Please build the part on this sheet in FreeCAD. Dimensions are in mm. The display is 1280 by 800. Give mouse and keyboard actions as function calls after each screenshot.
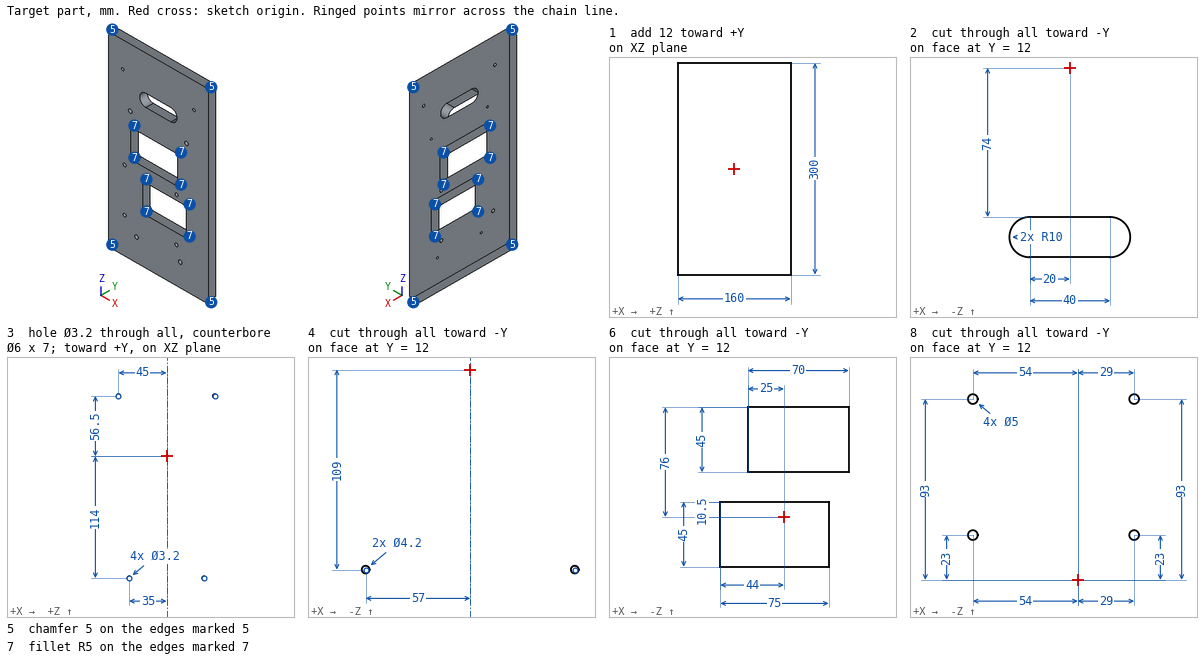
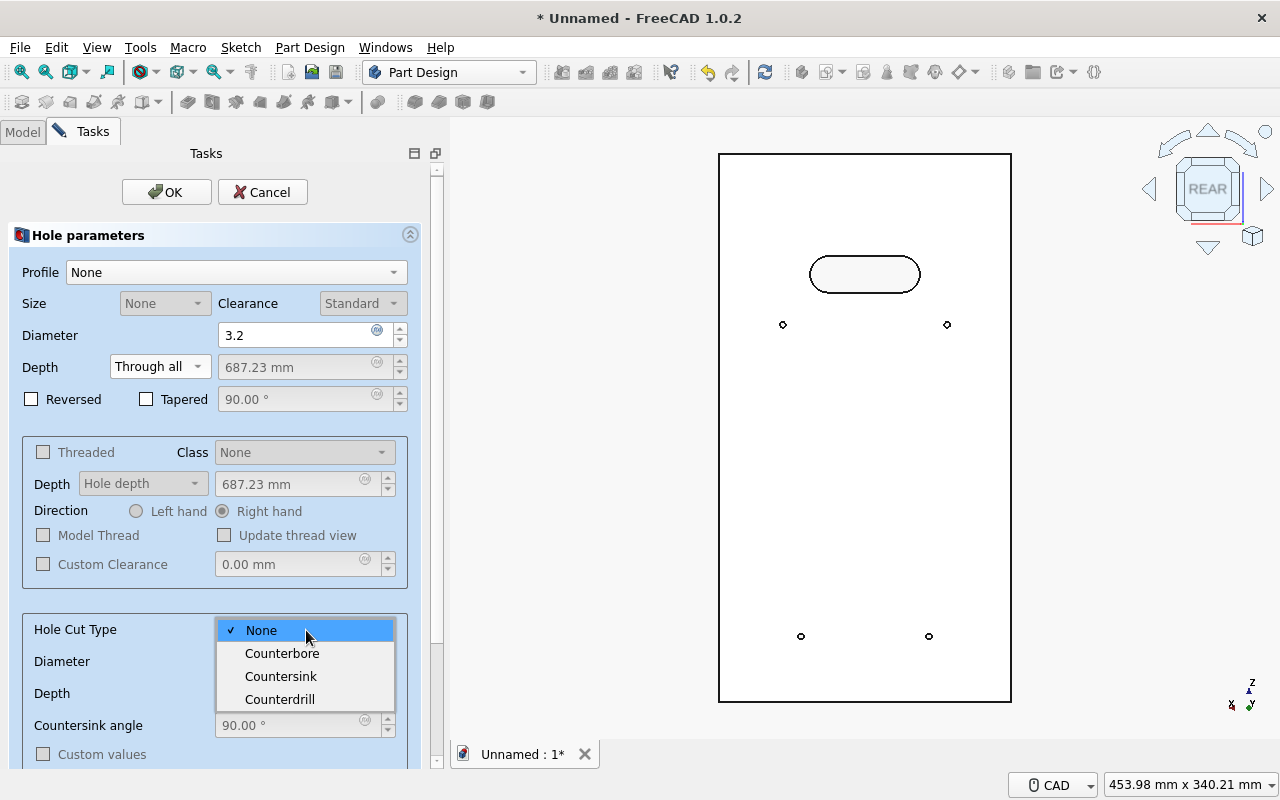
click(304, 654)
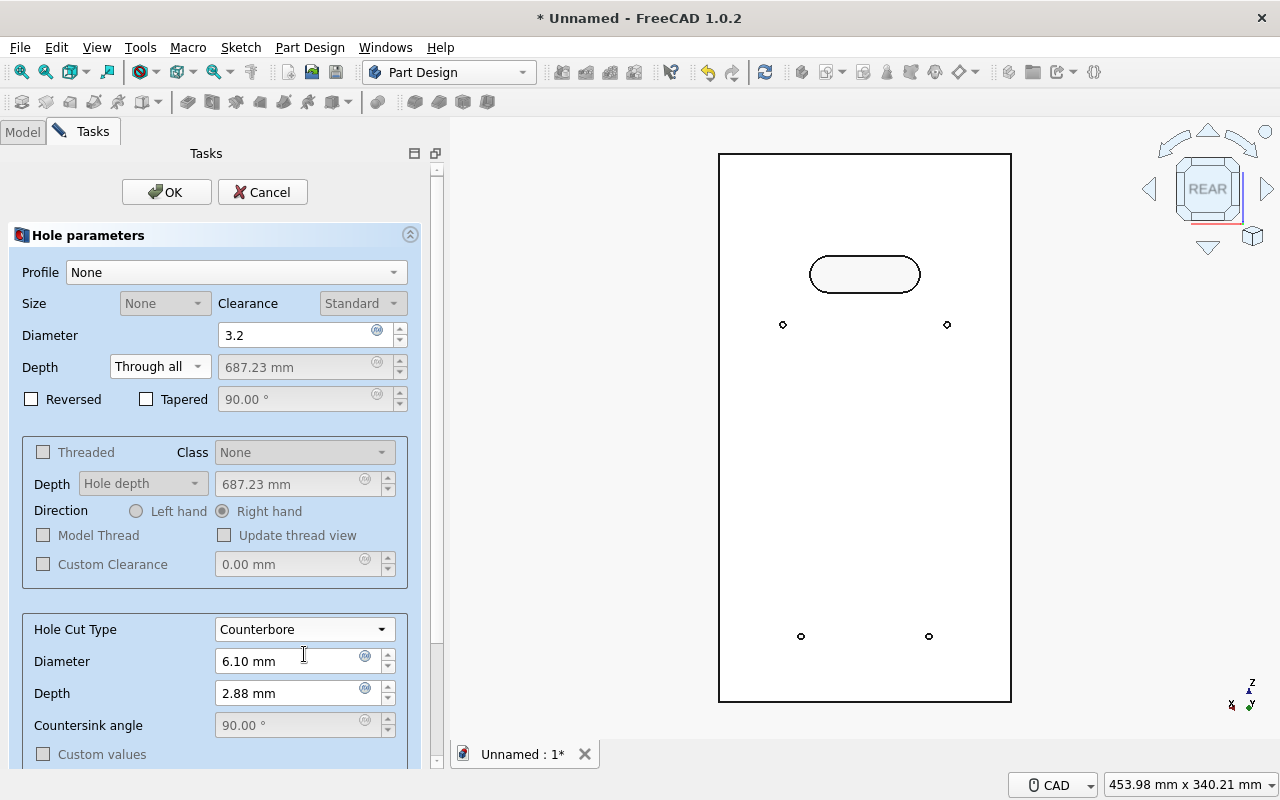
triple_click(298, 661)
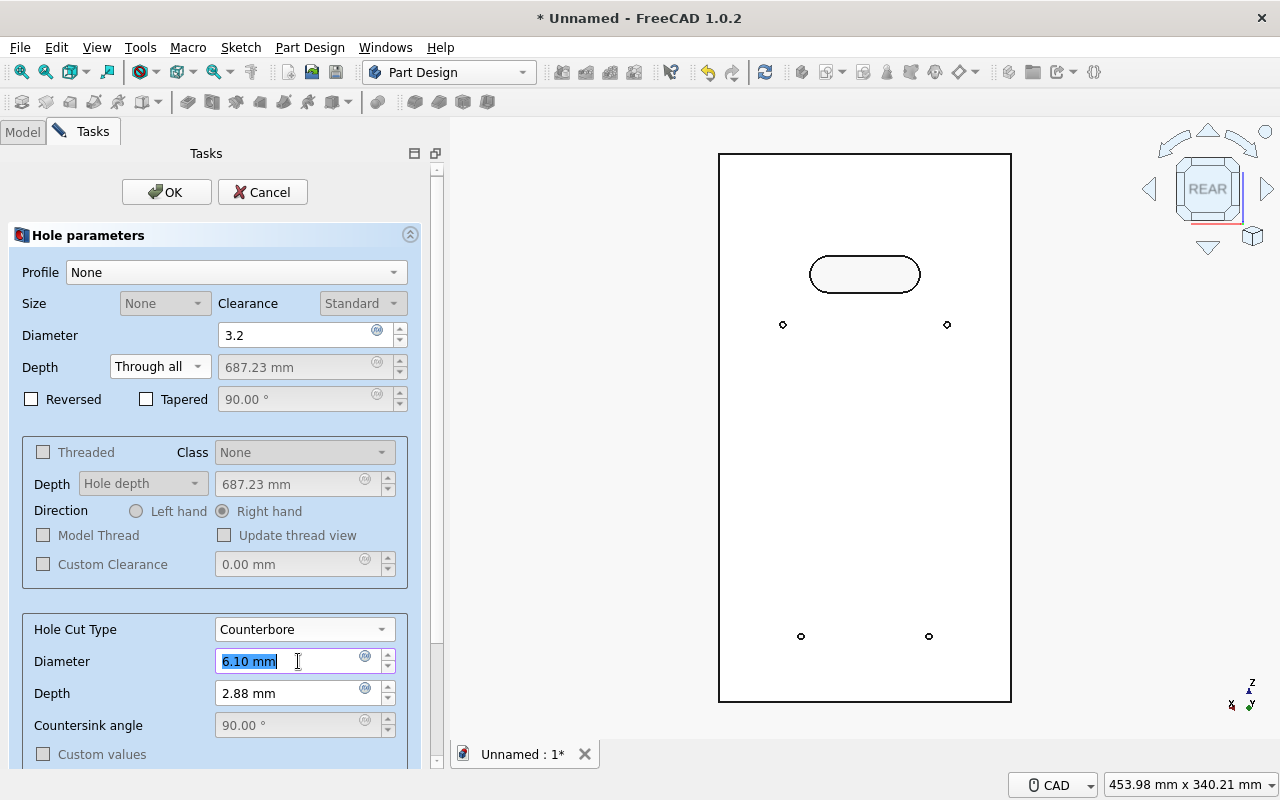
text(6)
key(Tab)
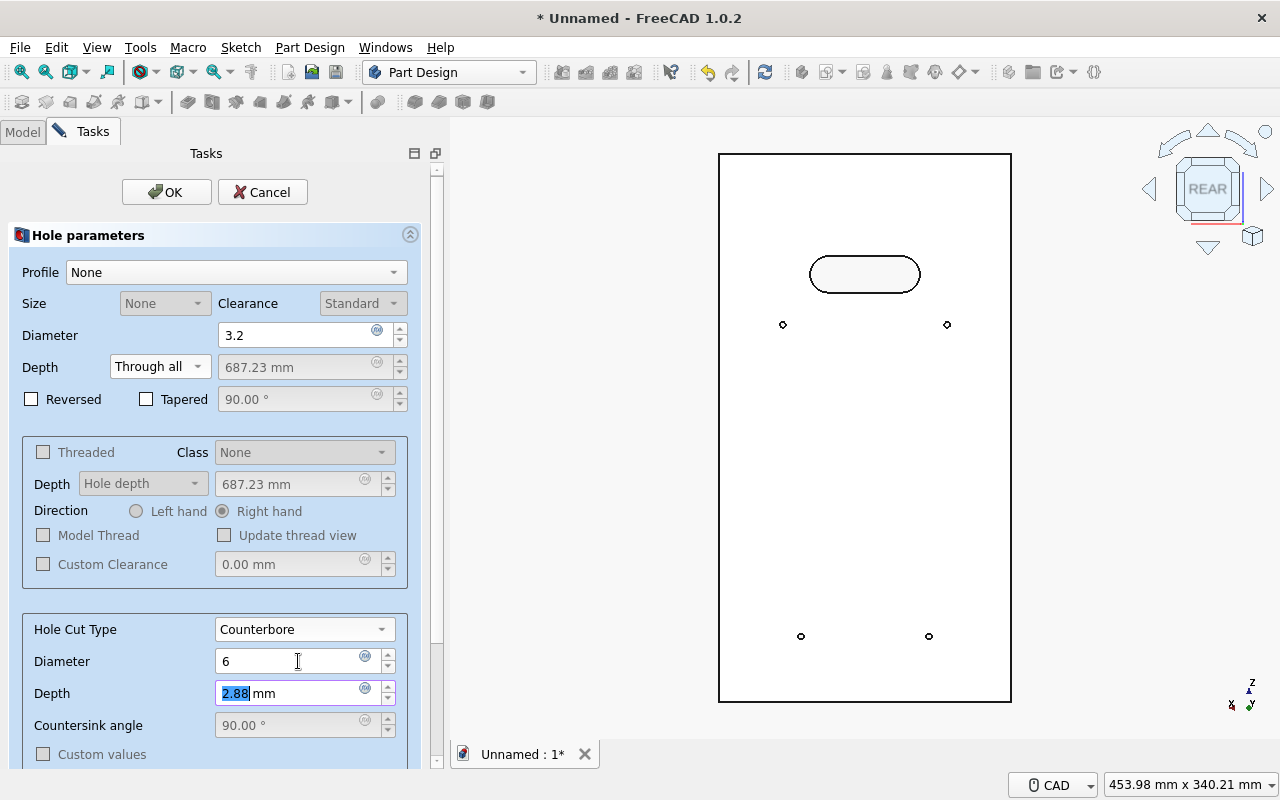
text(7)
key(Tab)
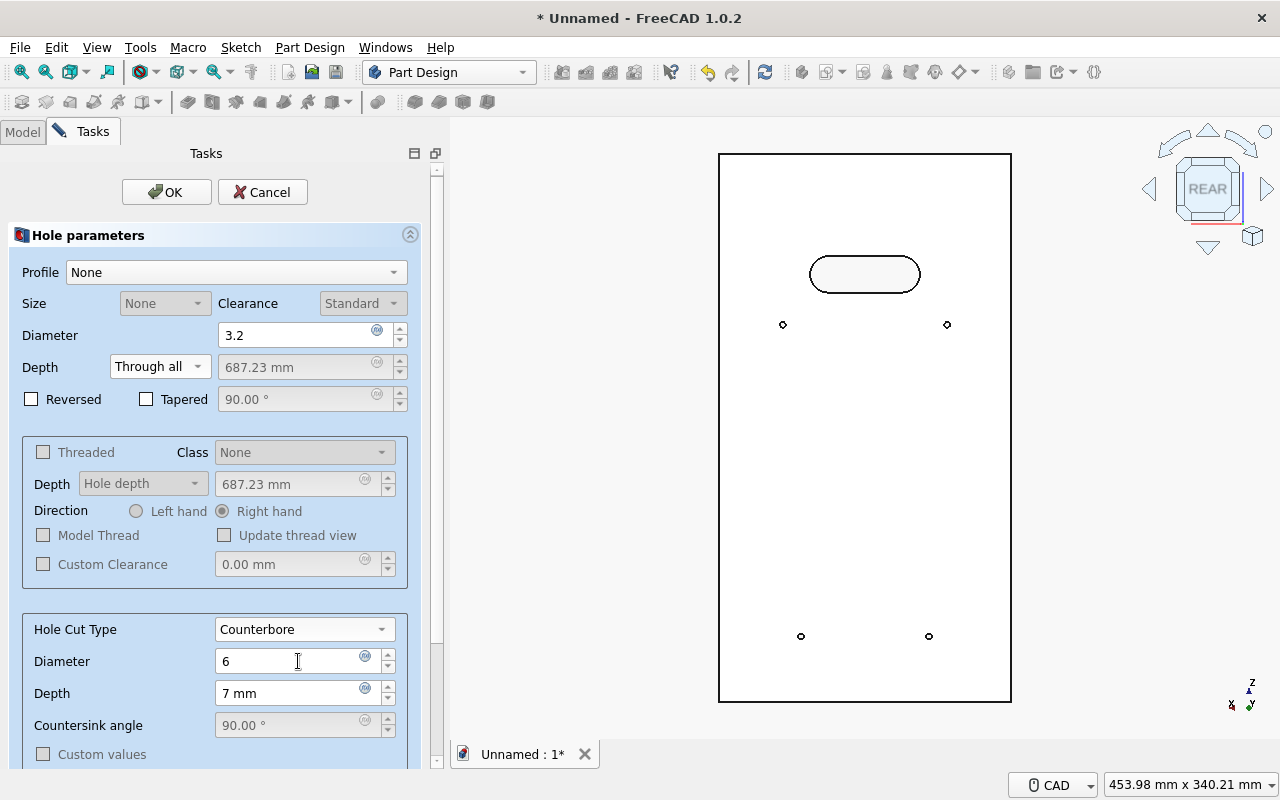
click(167, 192)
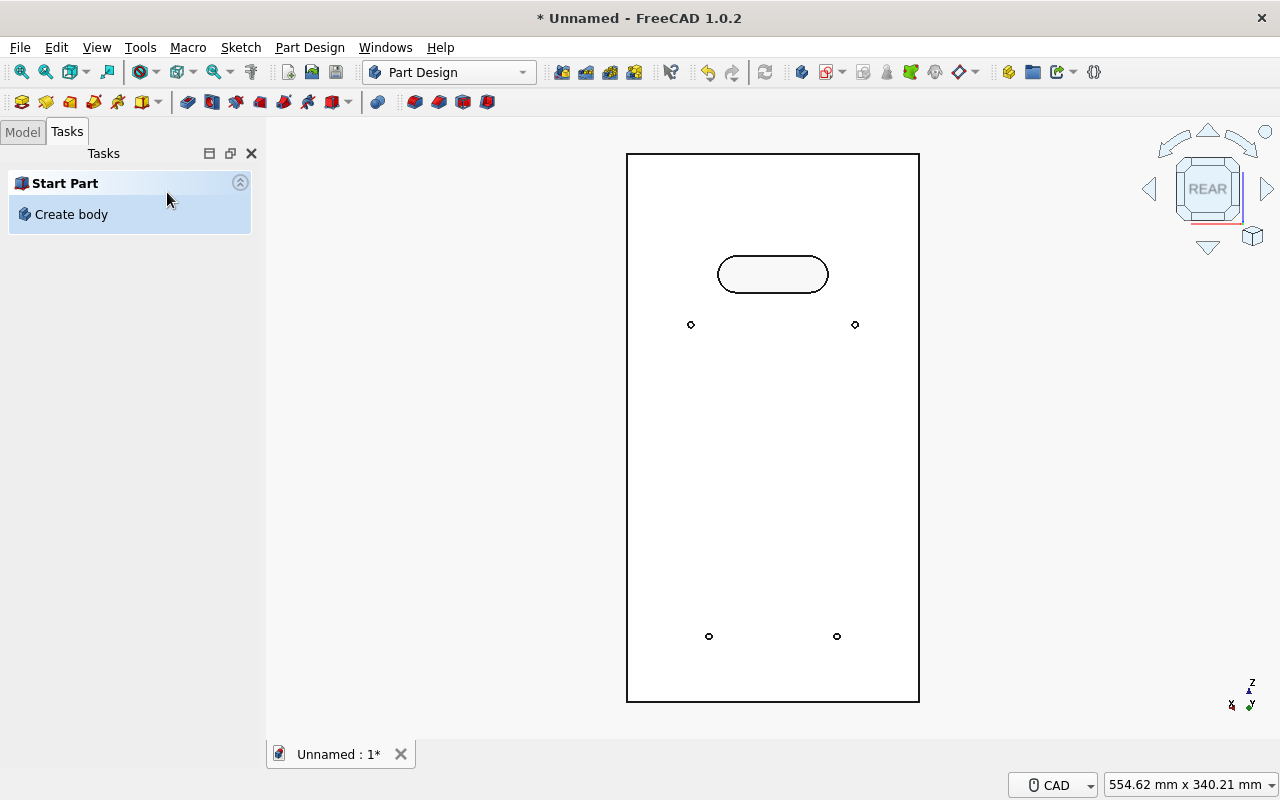
click(773, 505)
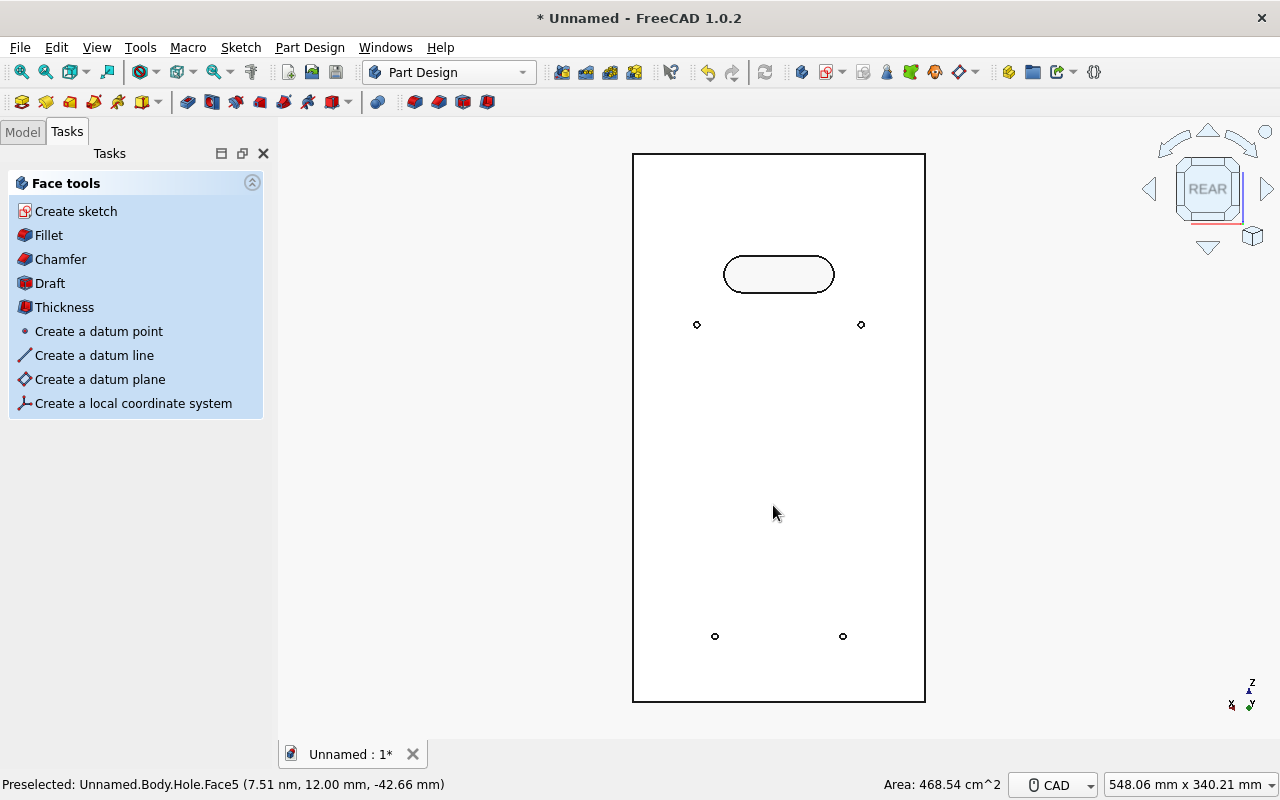
click(826, 72)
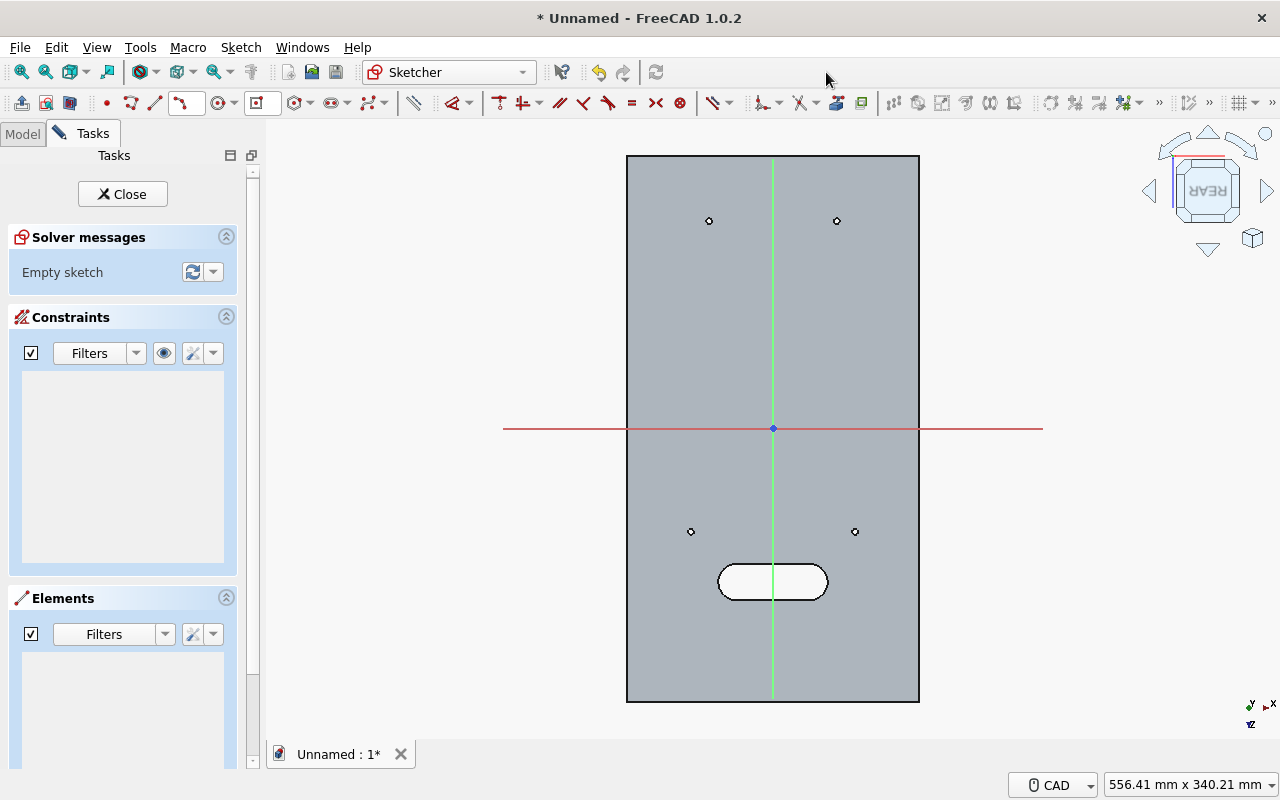
scroll(856, 653, up, 3)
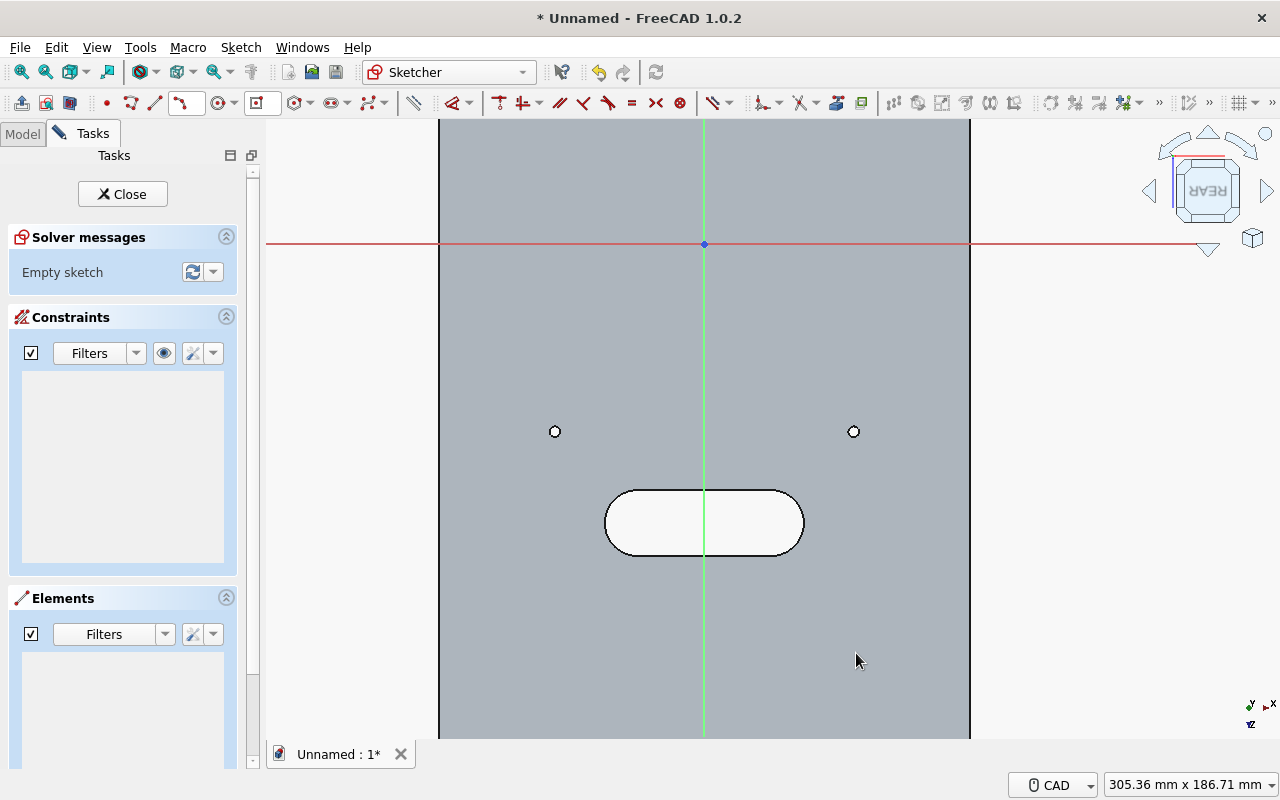
click(218, 104)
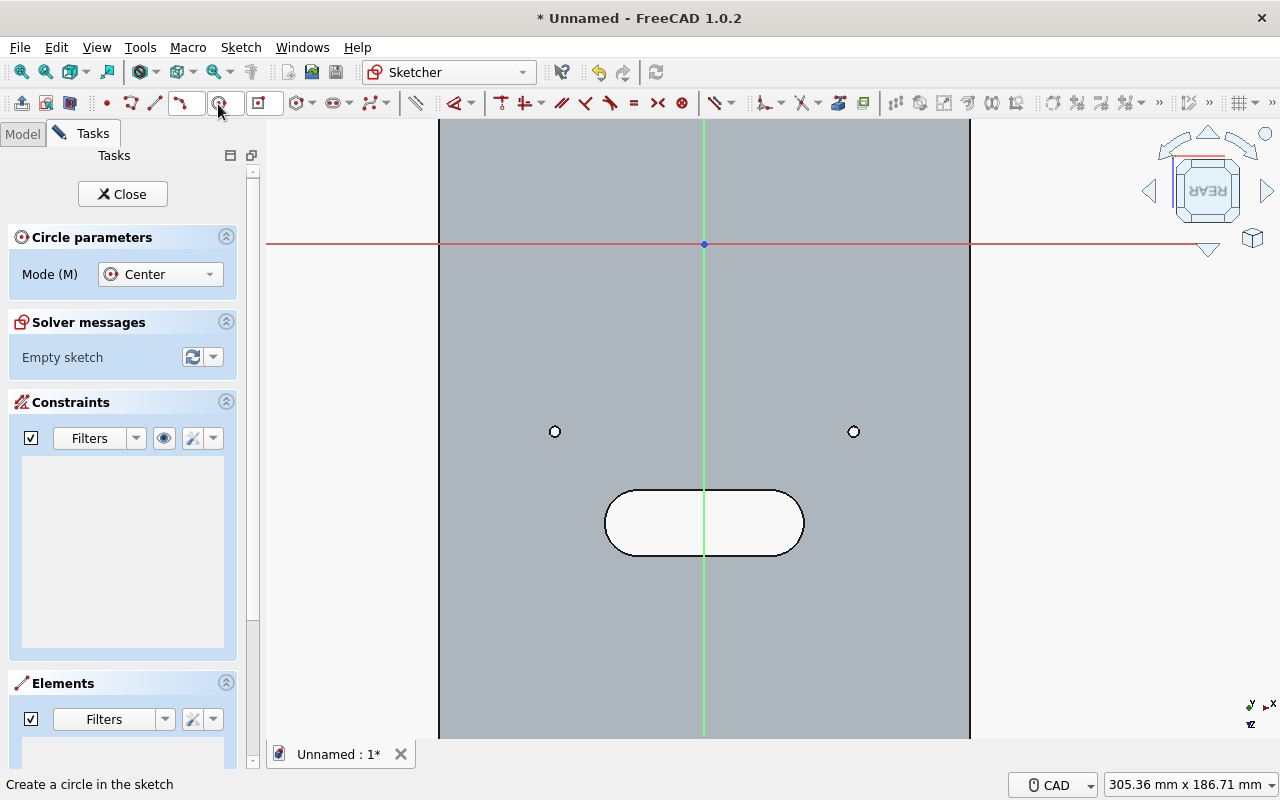
scroll(515, 606, up, 6)